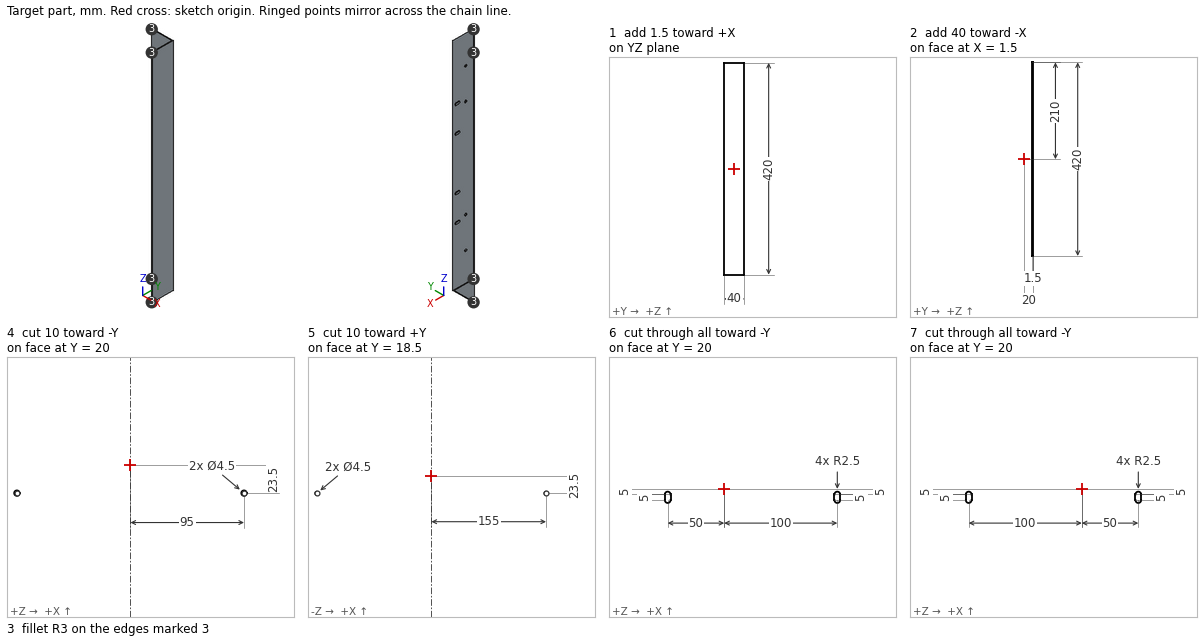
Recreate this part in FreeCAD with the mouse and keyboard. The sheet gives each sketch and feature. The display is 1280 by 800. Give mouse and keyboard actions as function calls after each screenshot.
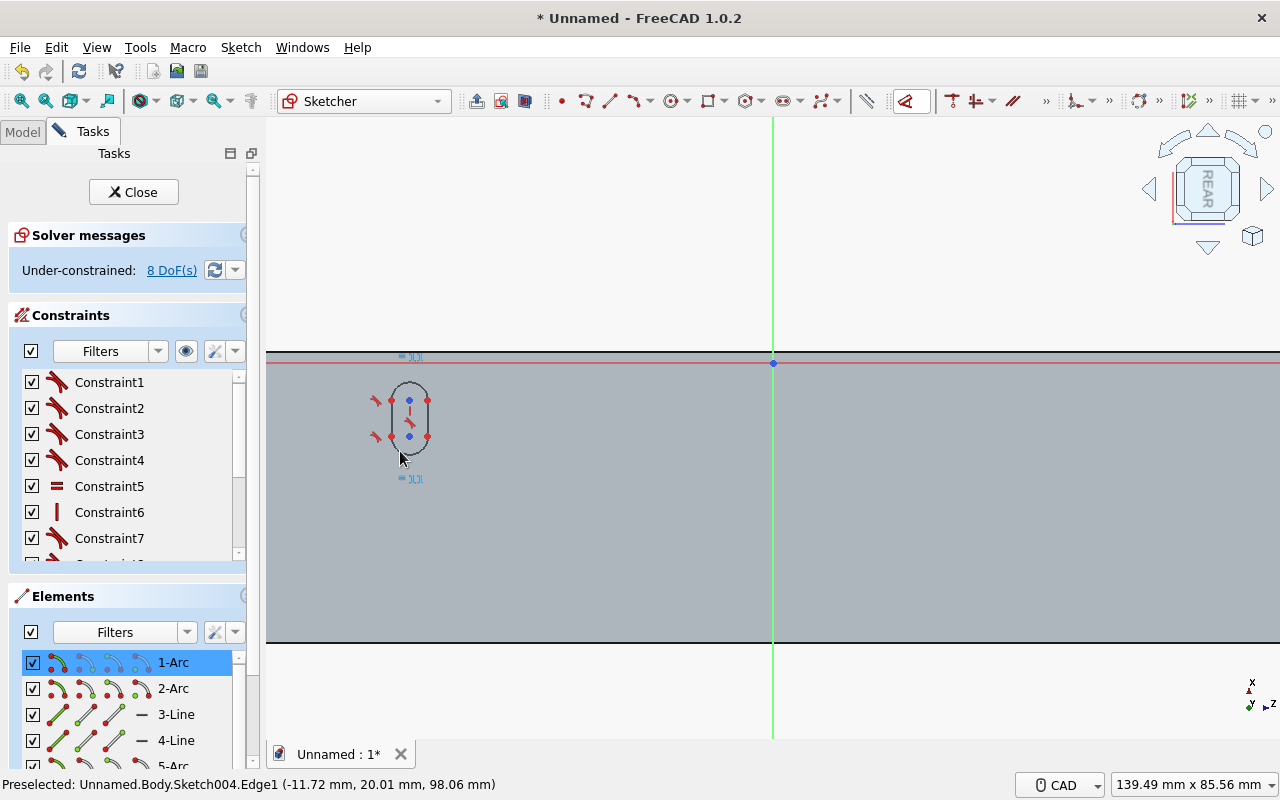
click(399, 451)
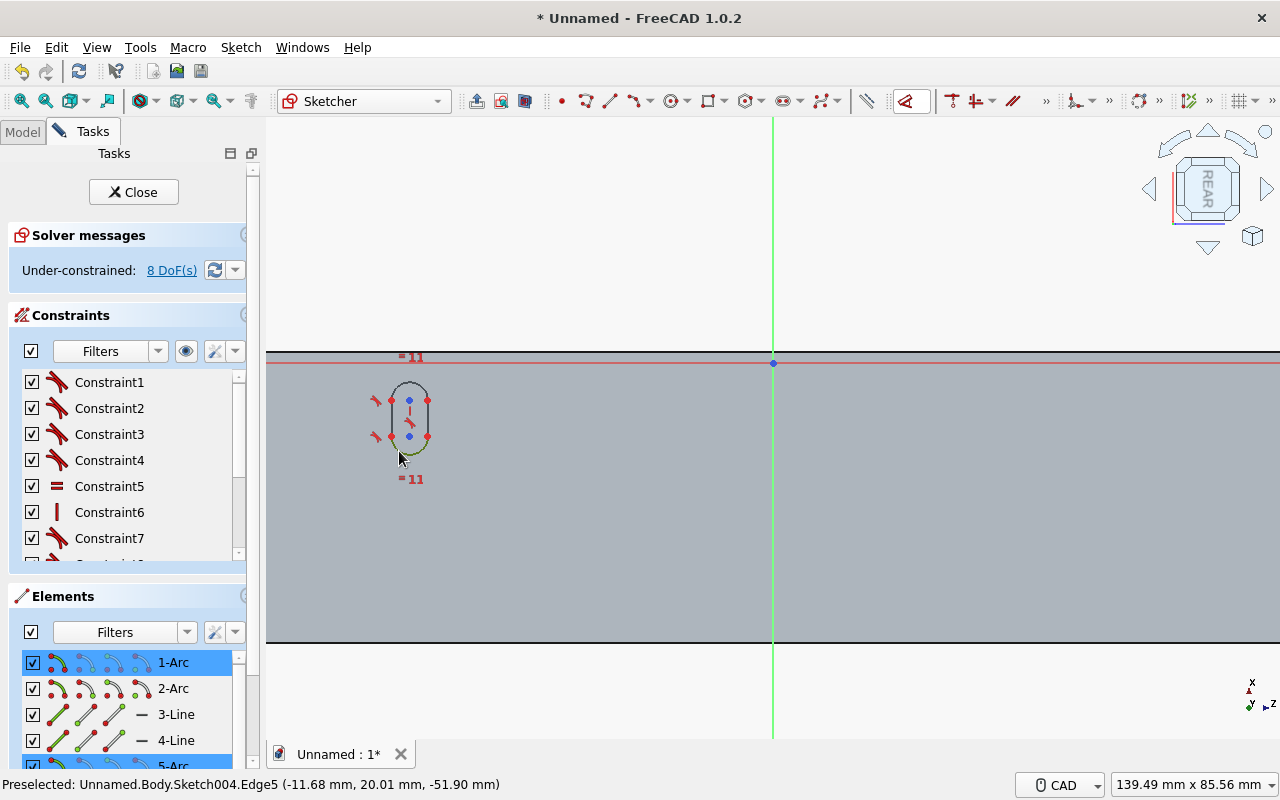
key(e)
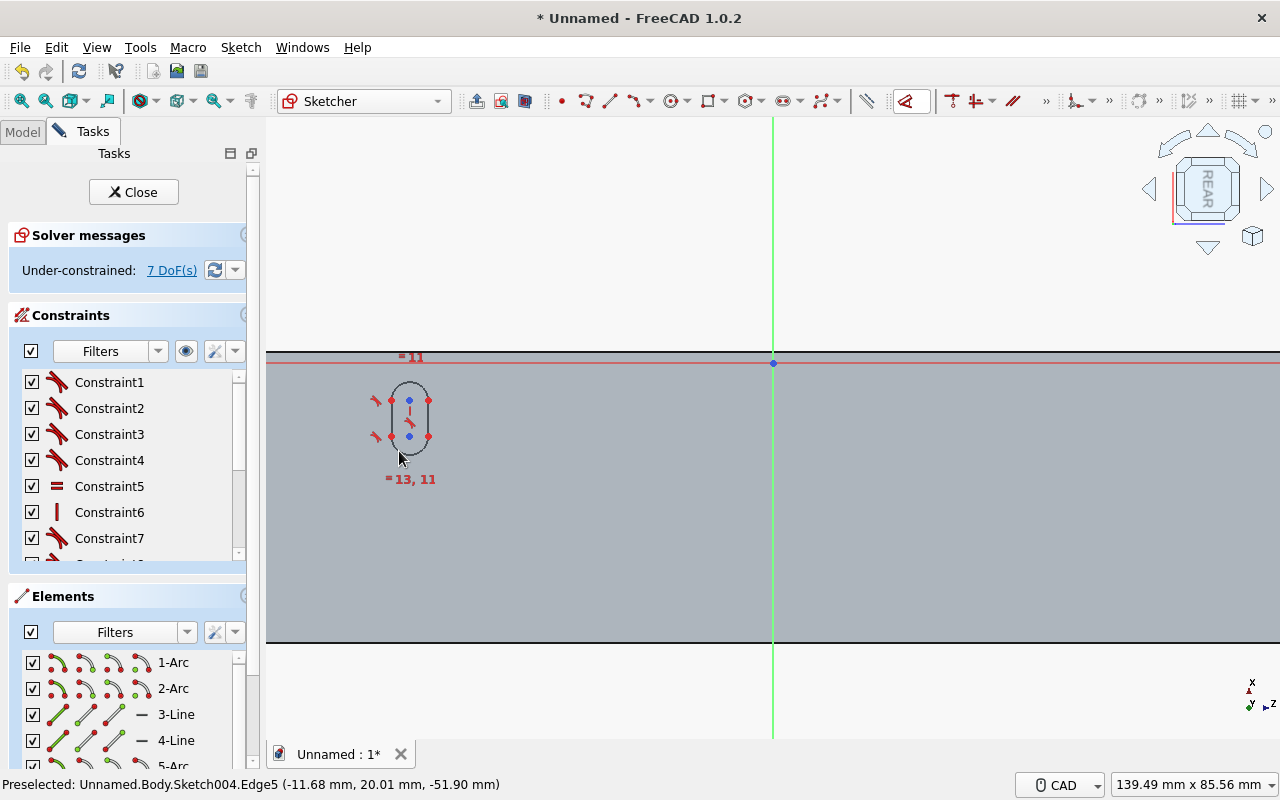
scroll(400, 451, down, 3)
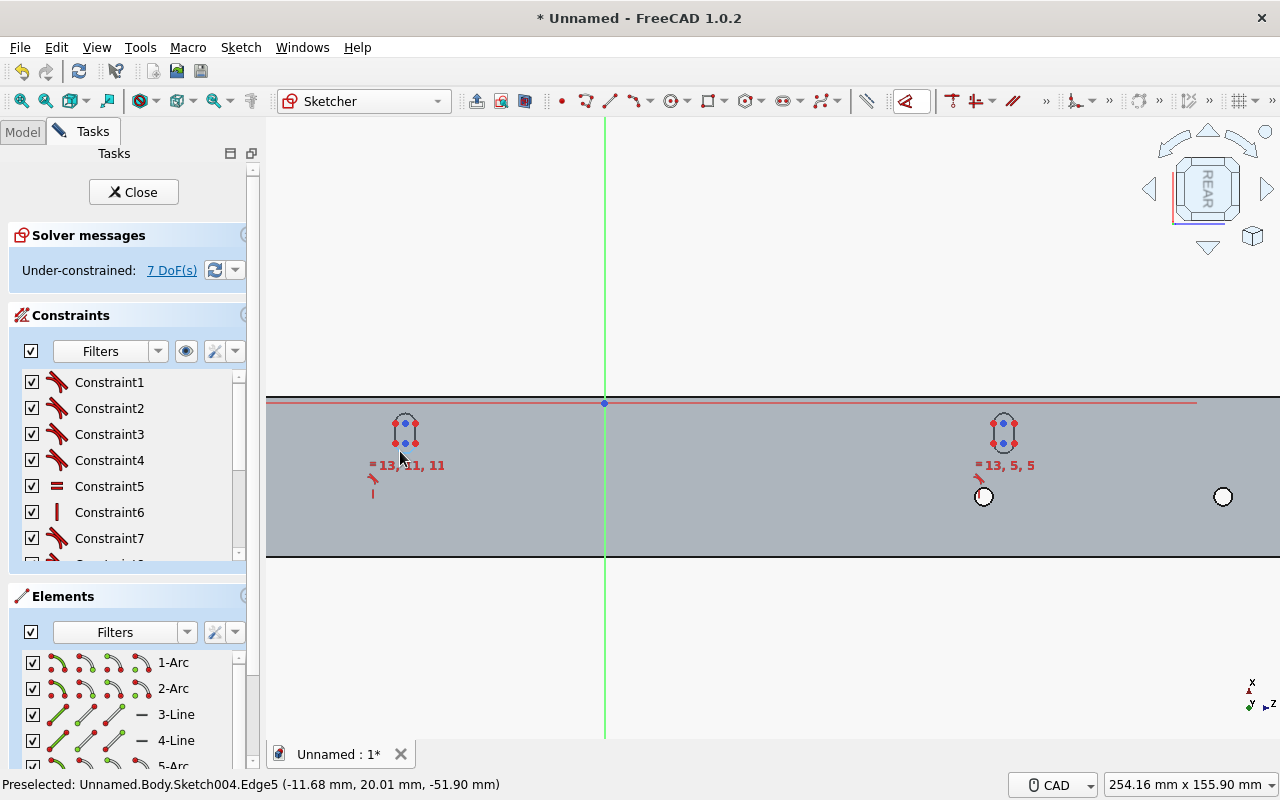
scroll(998, 451, up, 7)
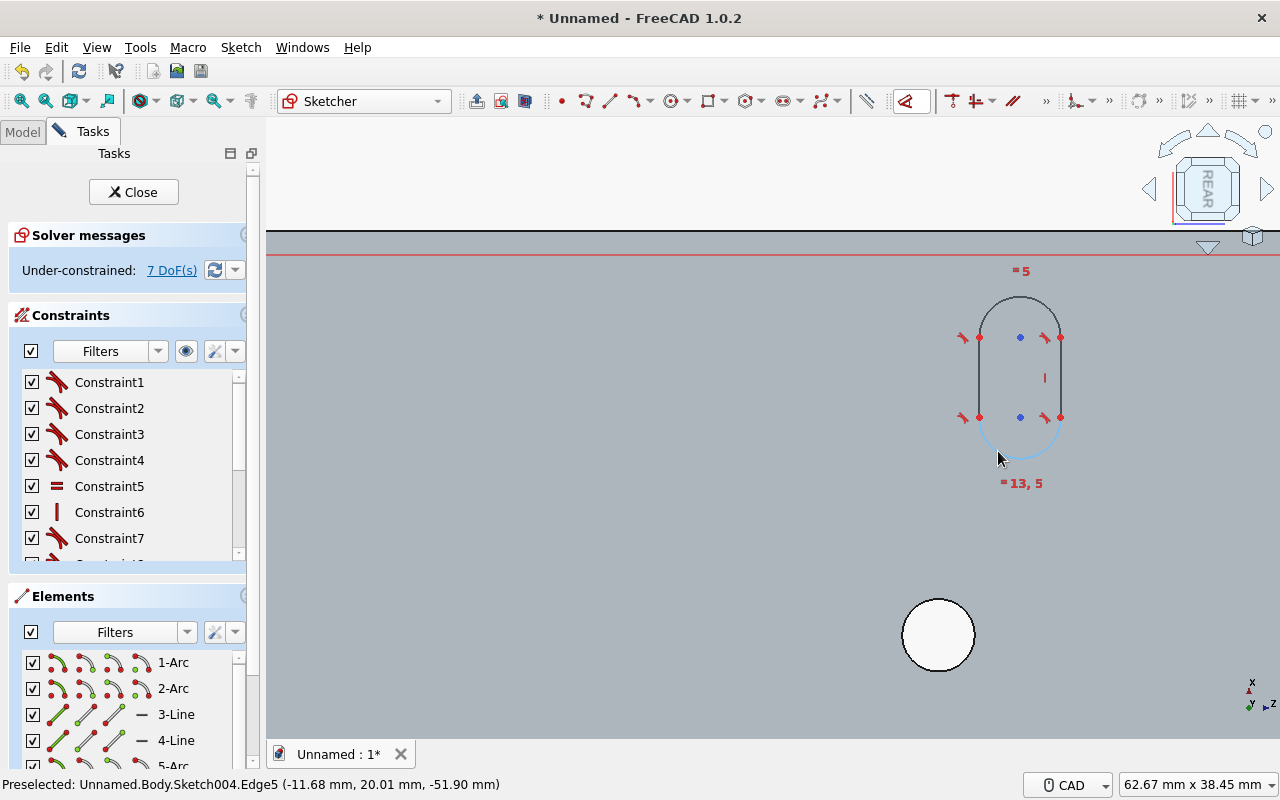
click(996, 451)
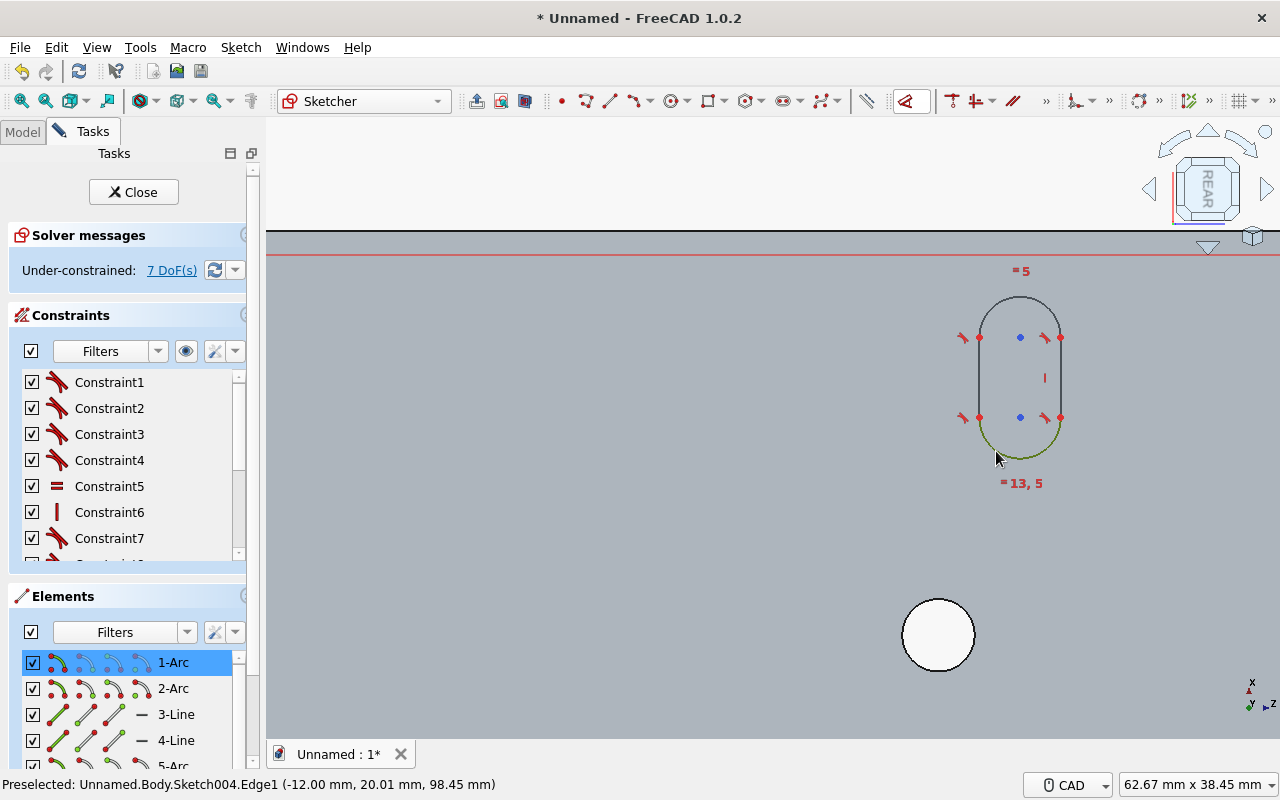
key(k)
key(r)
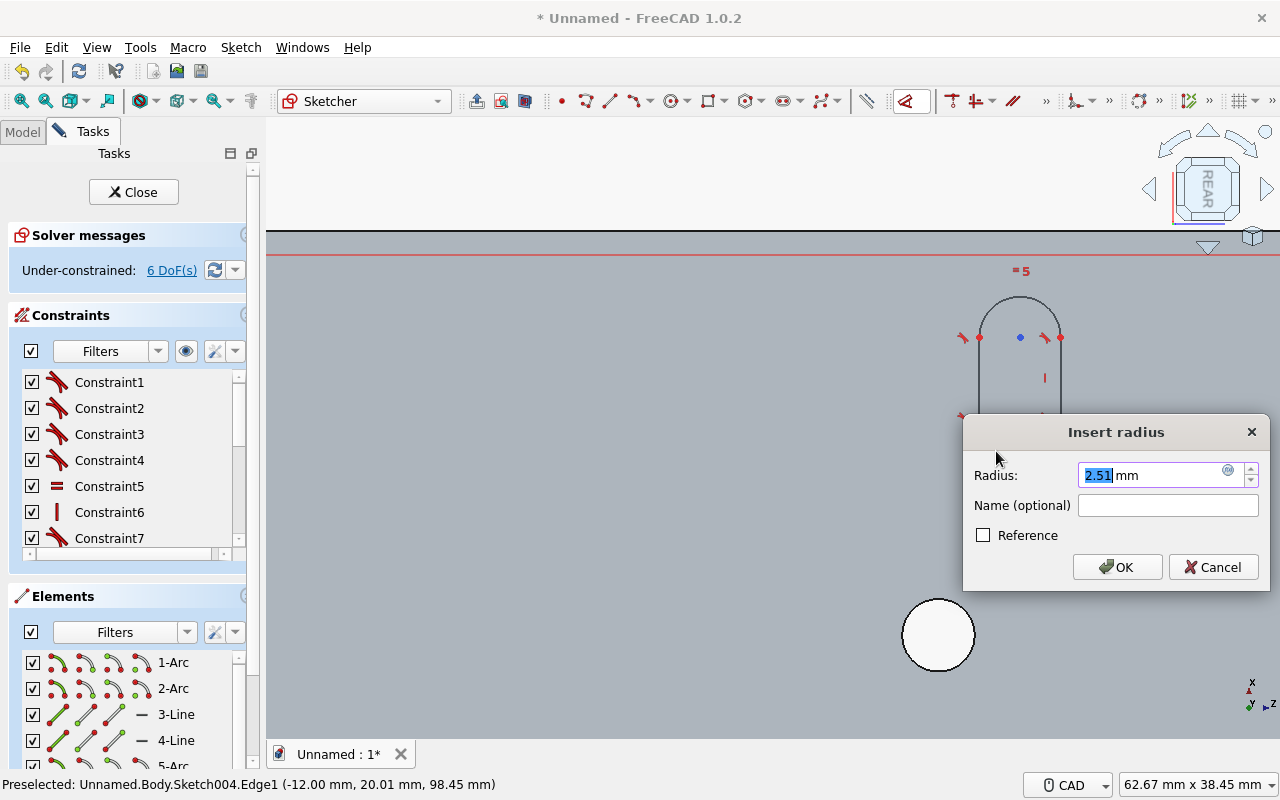
text(2.5)
key(Return)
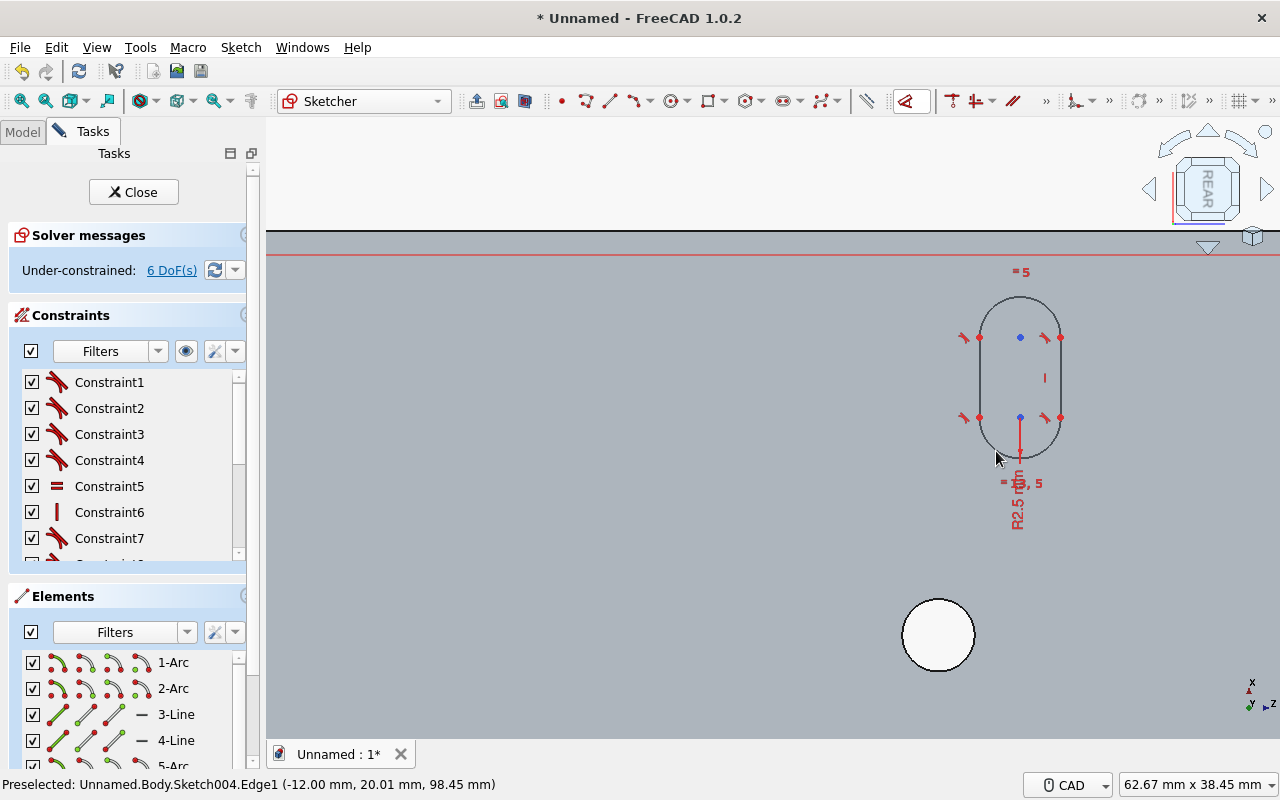
click(980, 394)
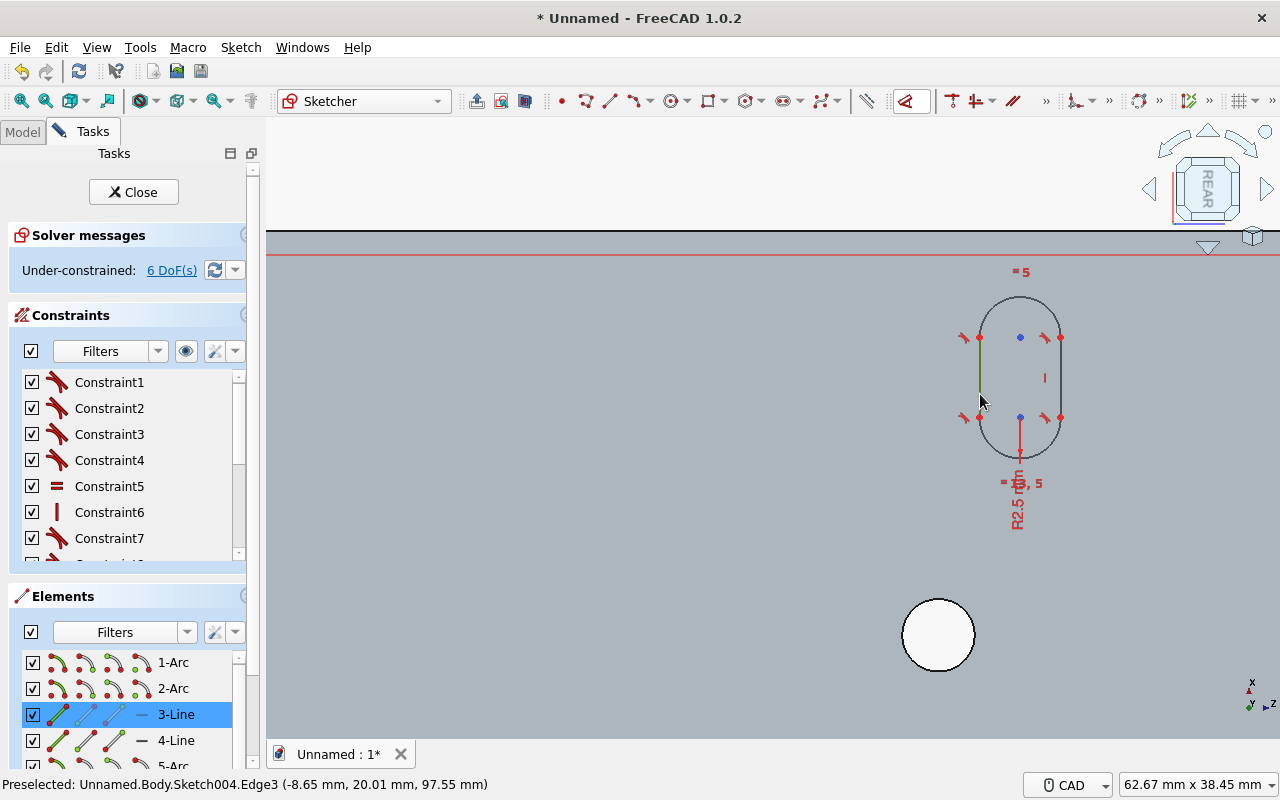
key(i)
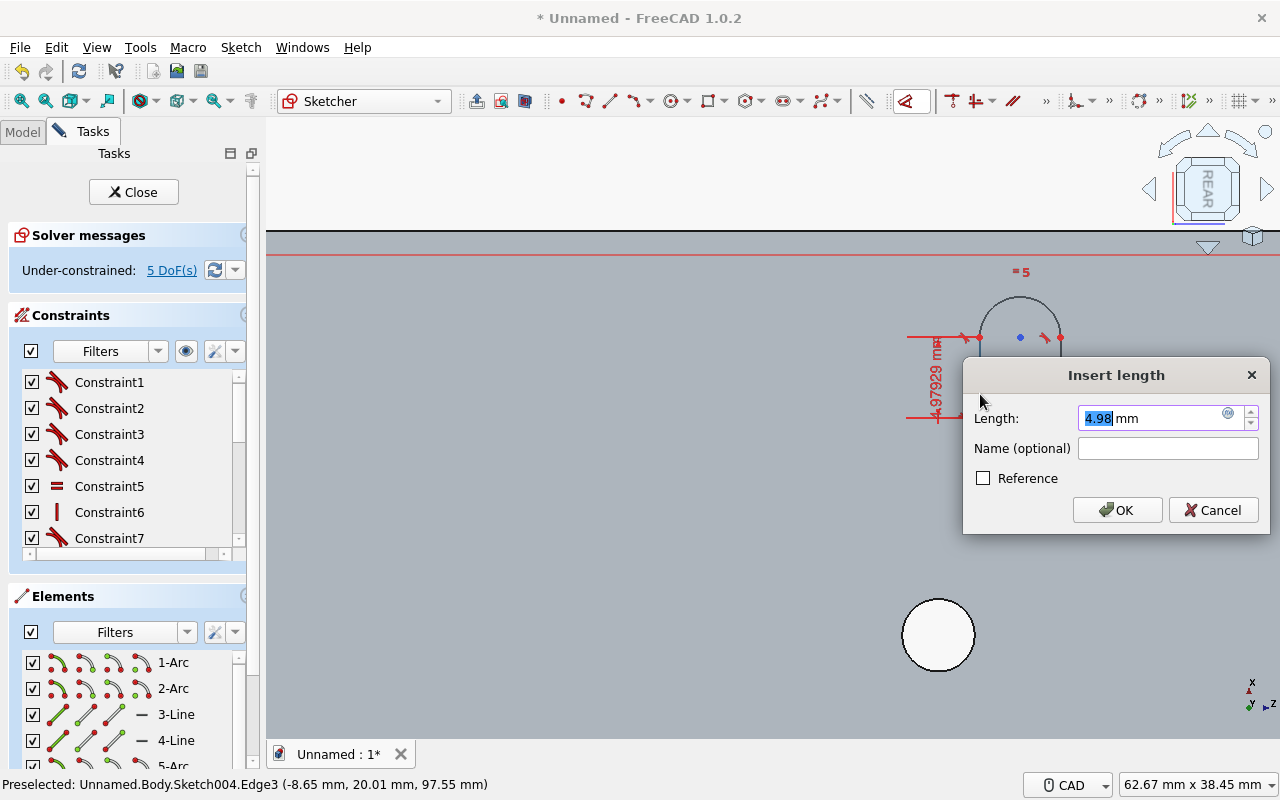
text(5)
key(Return)